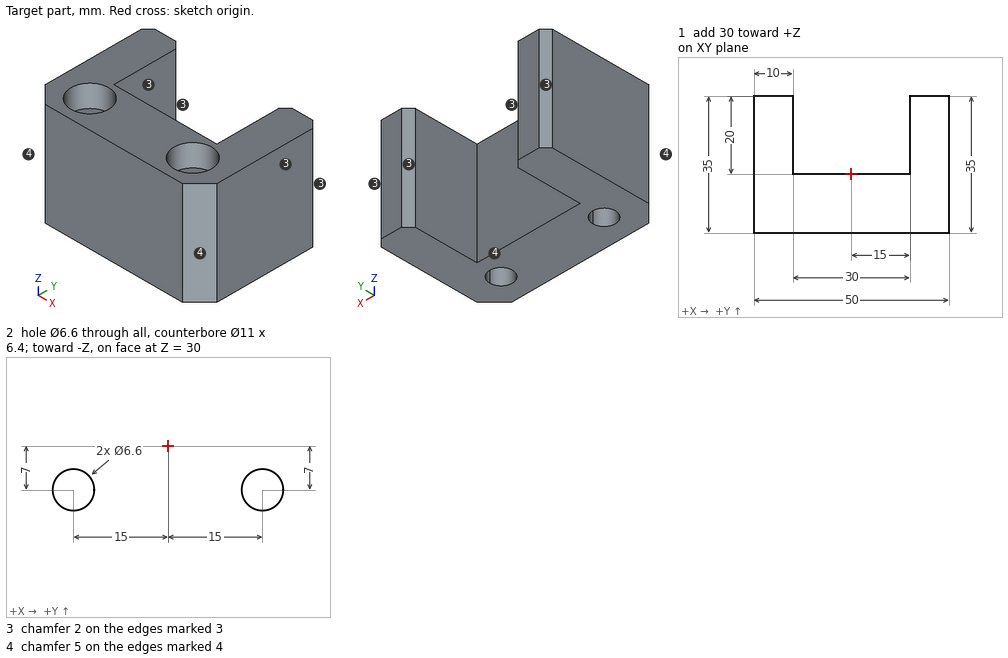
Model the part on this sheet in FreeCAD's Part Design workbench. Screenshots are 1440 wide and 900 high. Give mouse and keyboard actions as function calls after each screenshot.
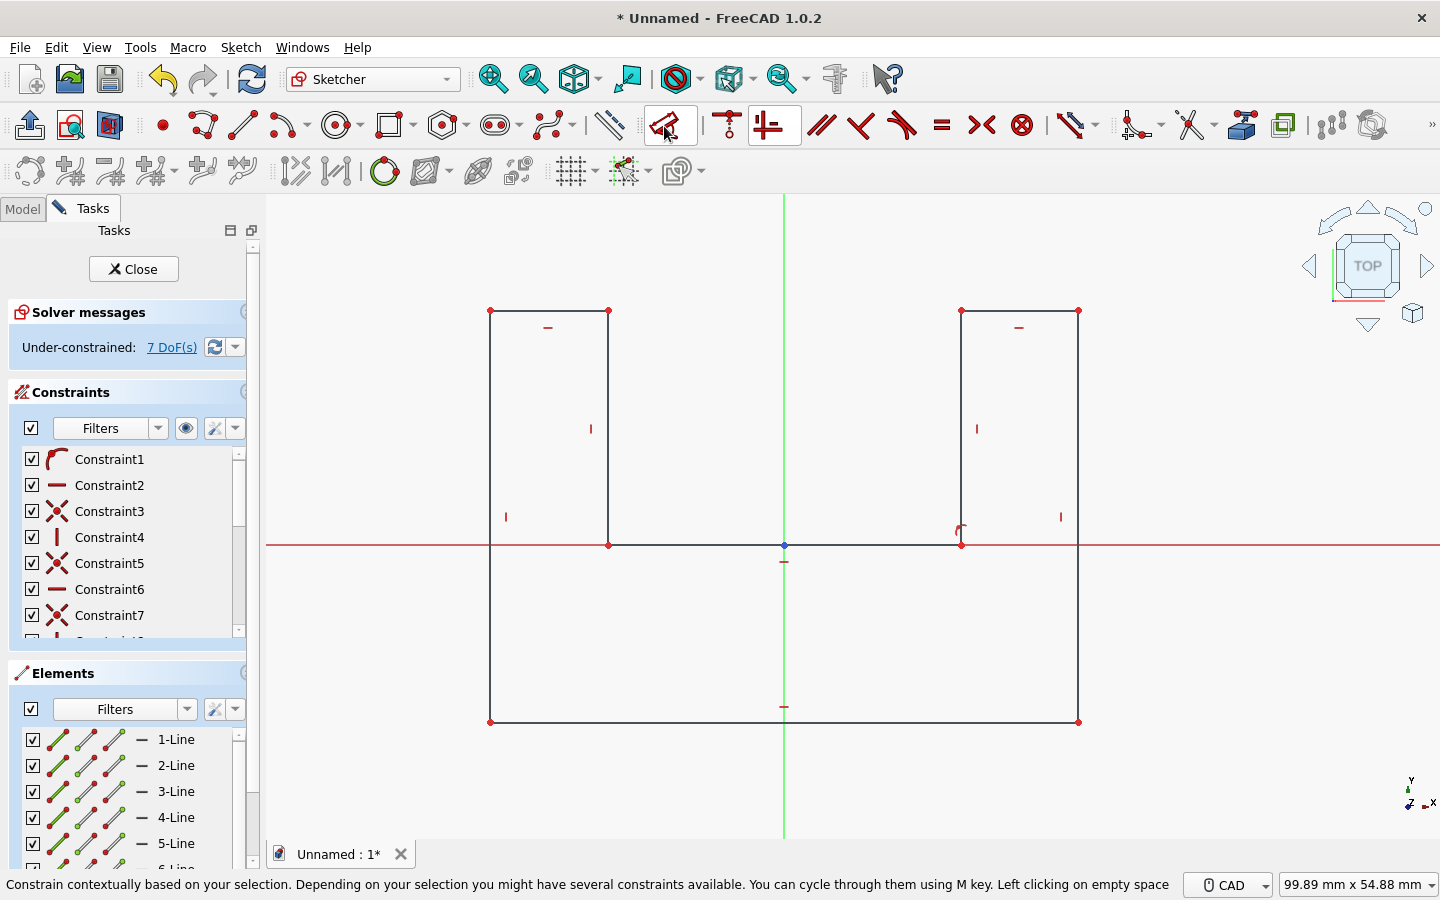
click(855, 545)
click(703, 579)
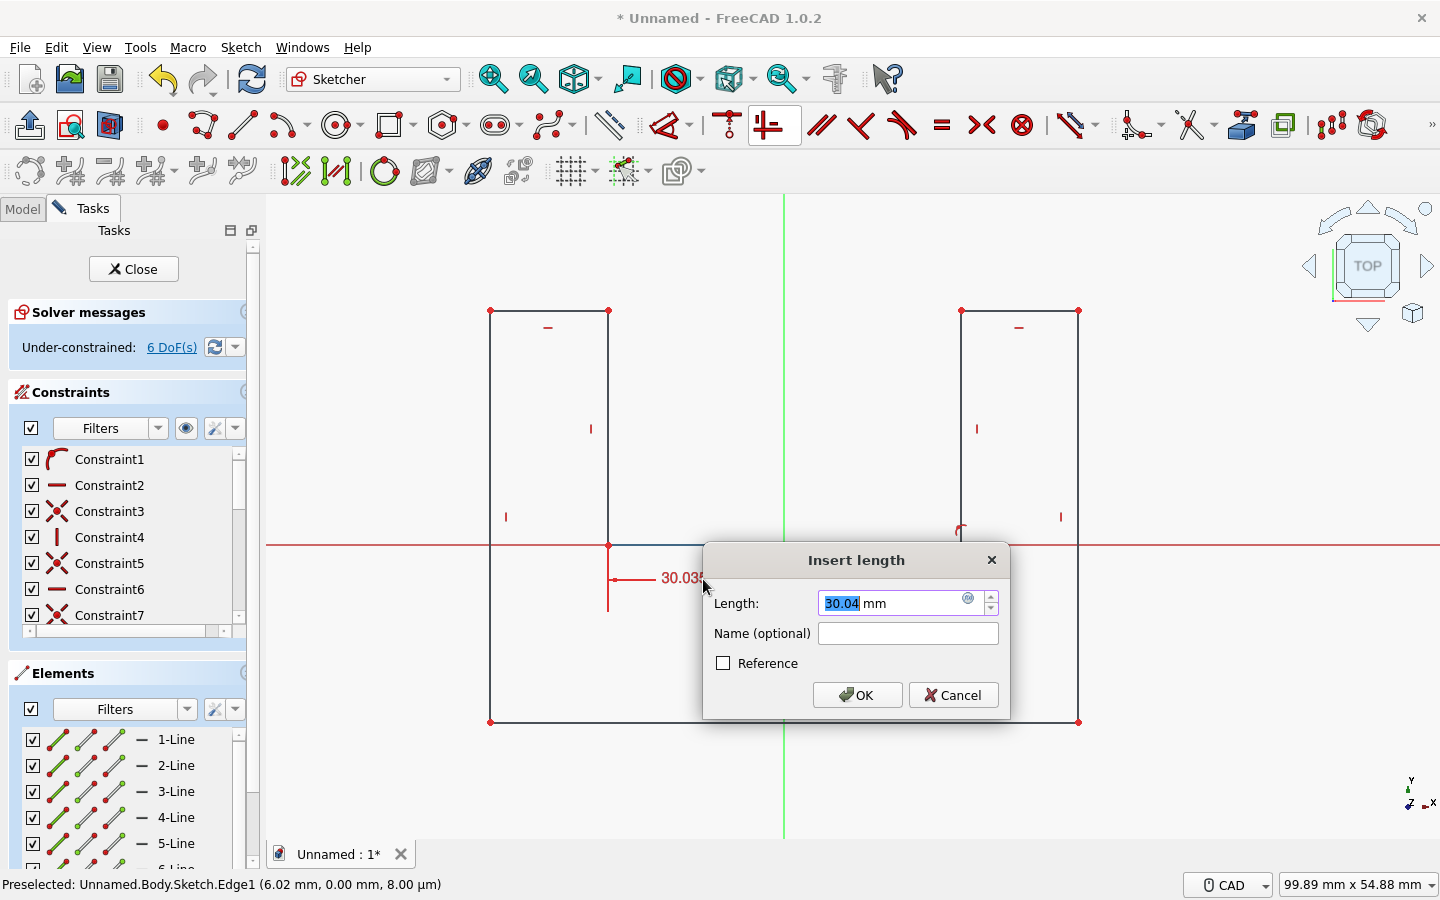
text(30)
key(Return)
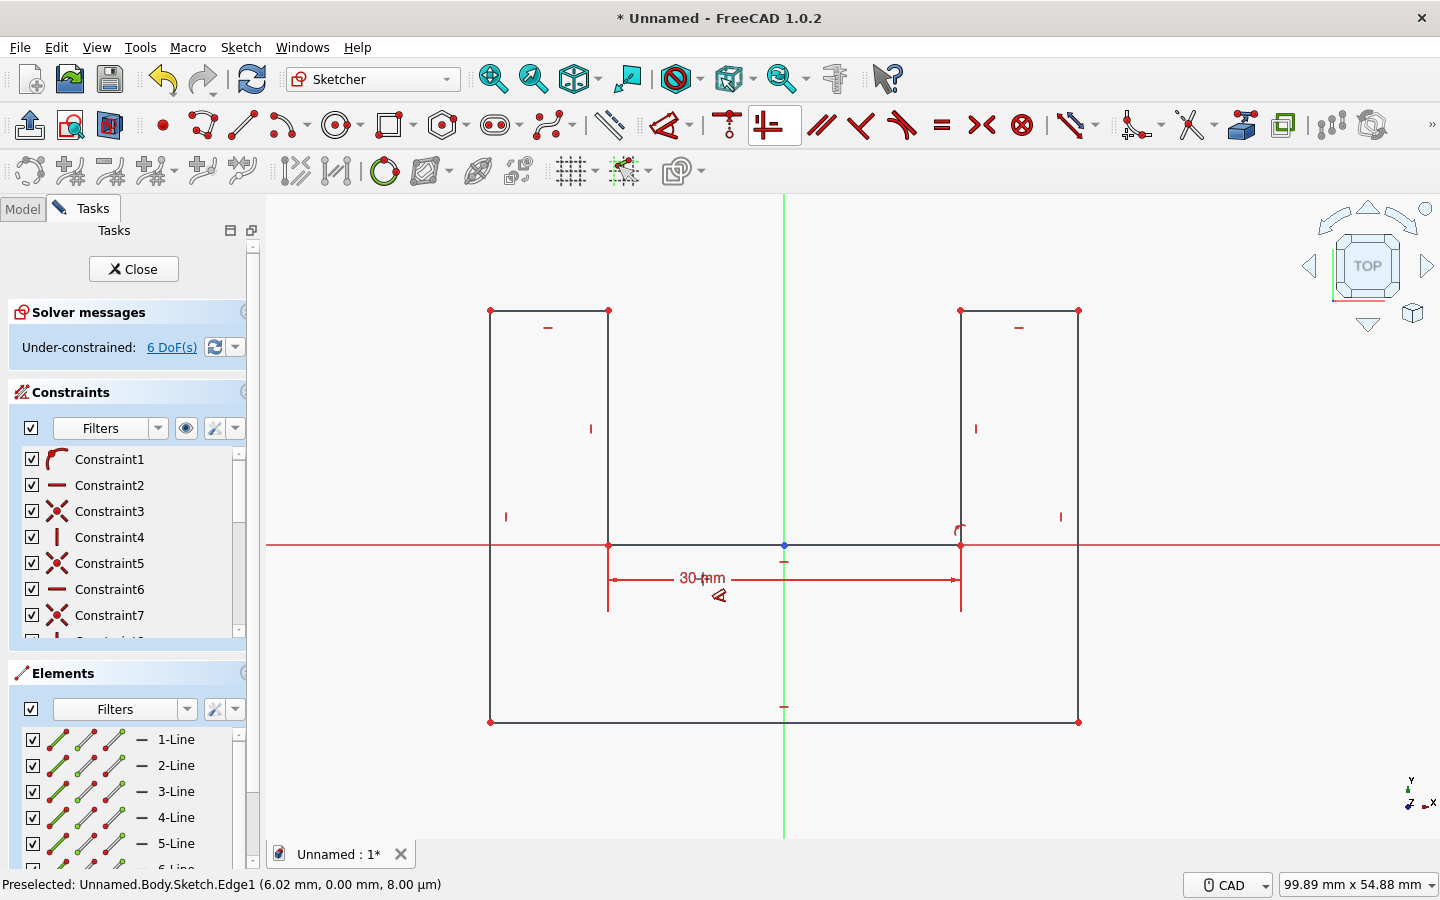
click(608, 475)
click(574, 428)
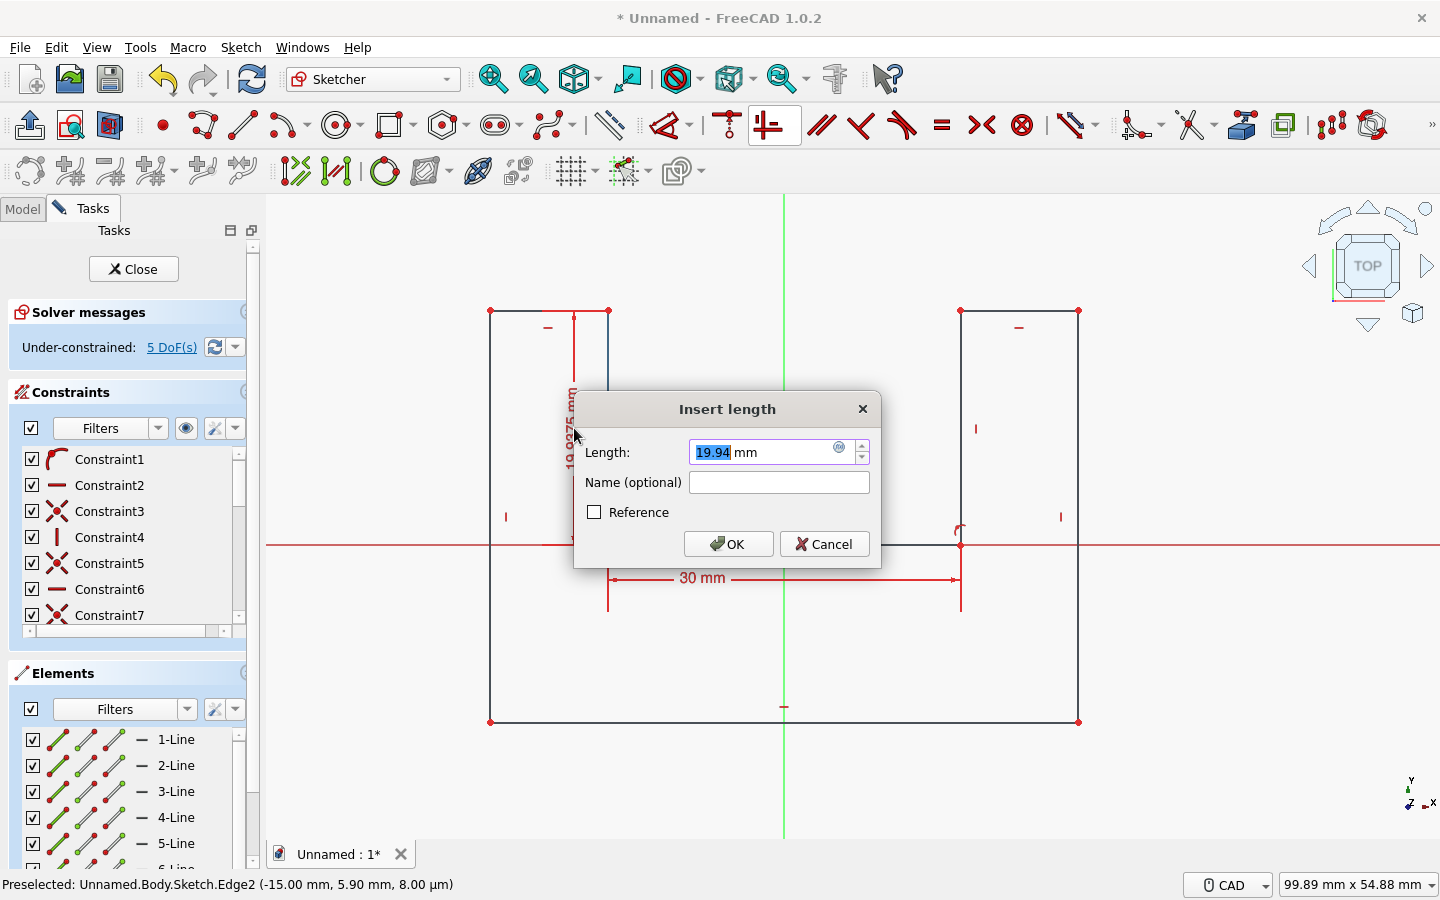
text(20)
key(Return)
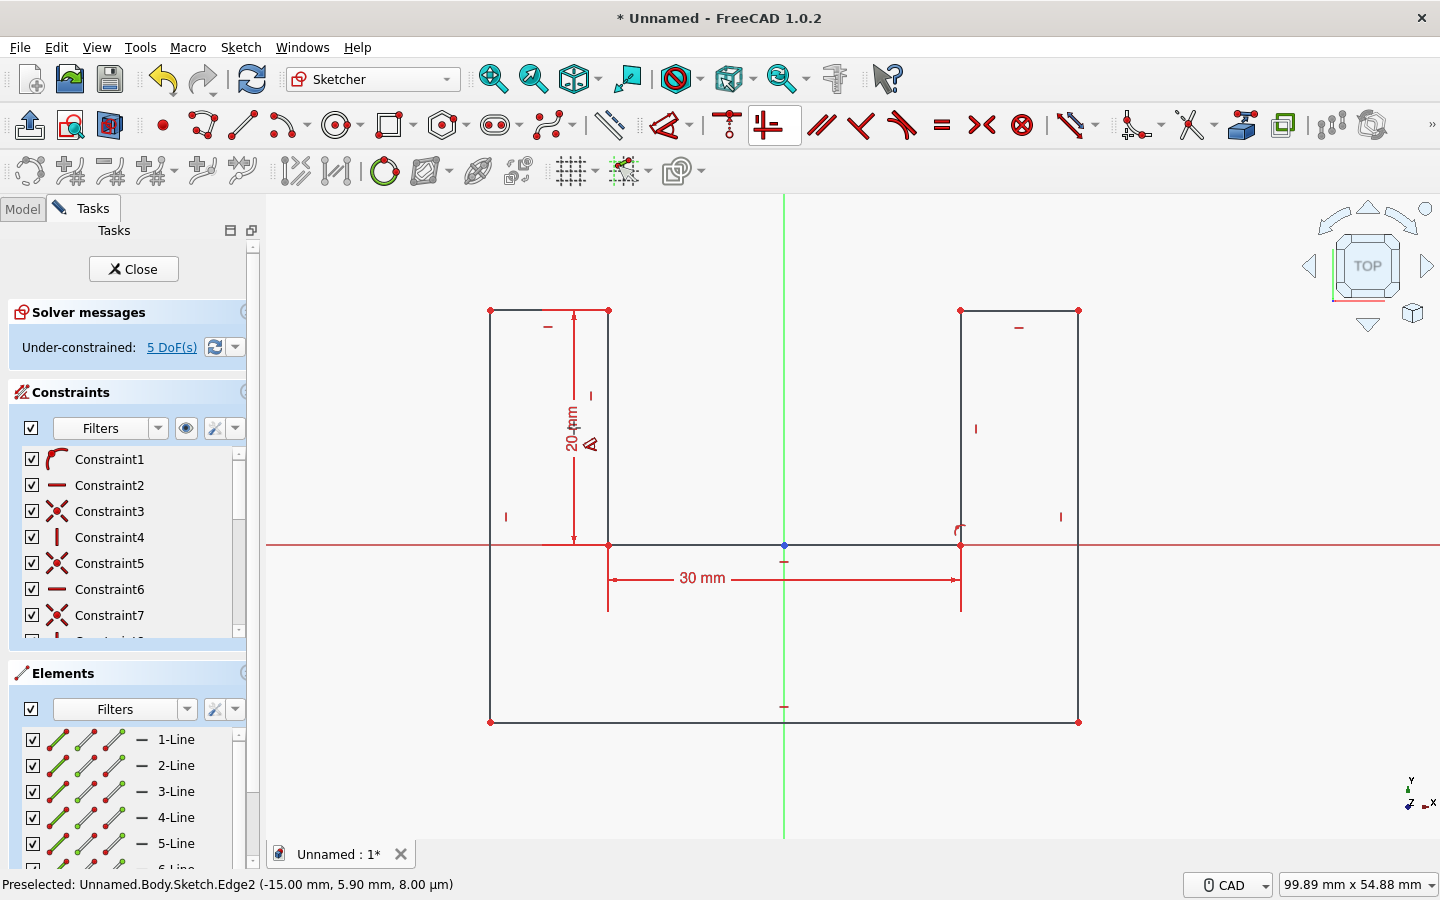
click(573, 310)
click(549, 276)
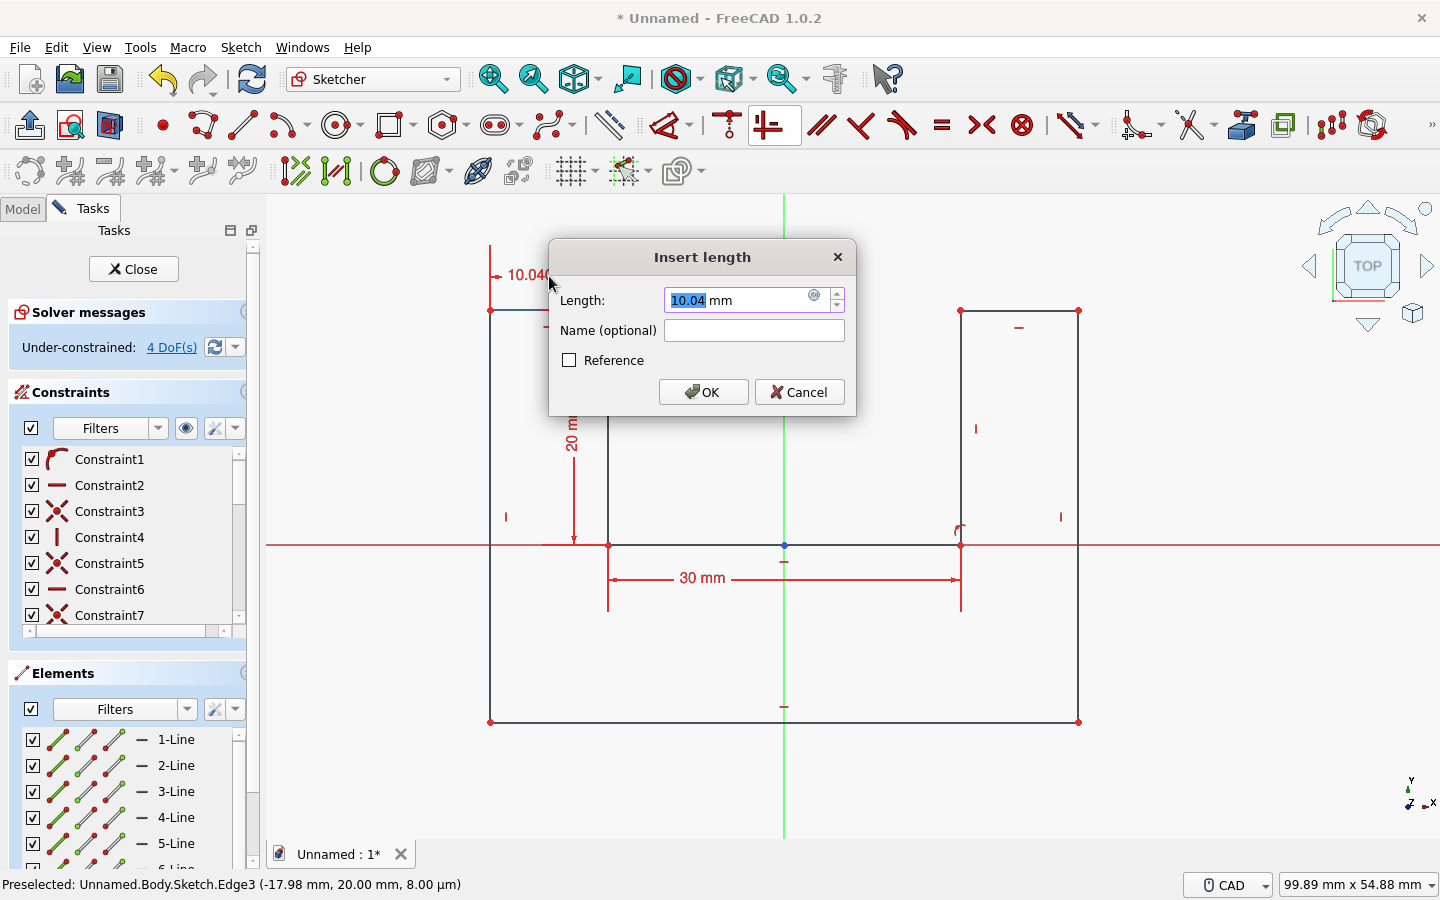
text(10)
key(Return)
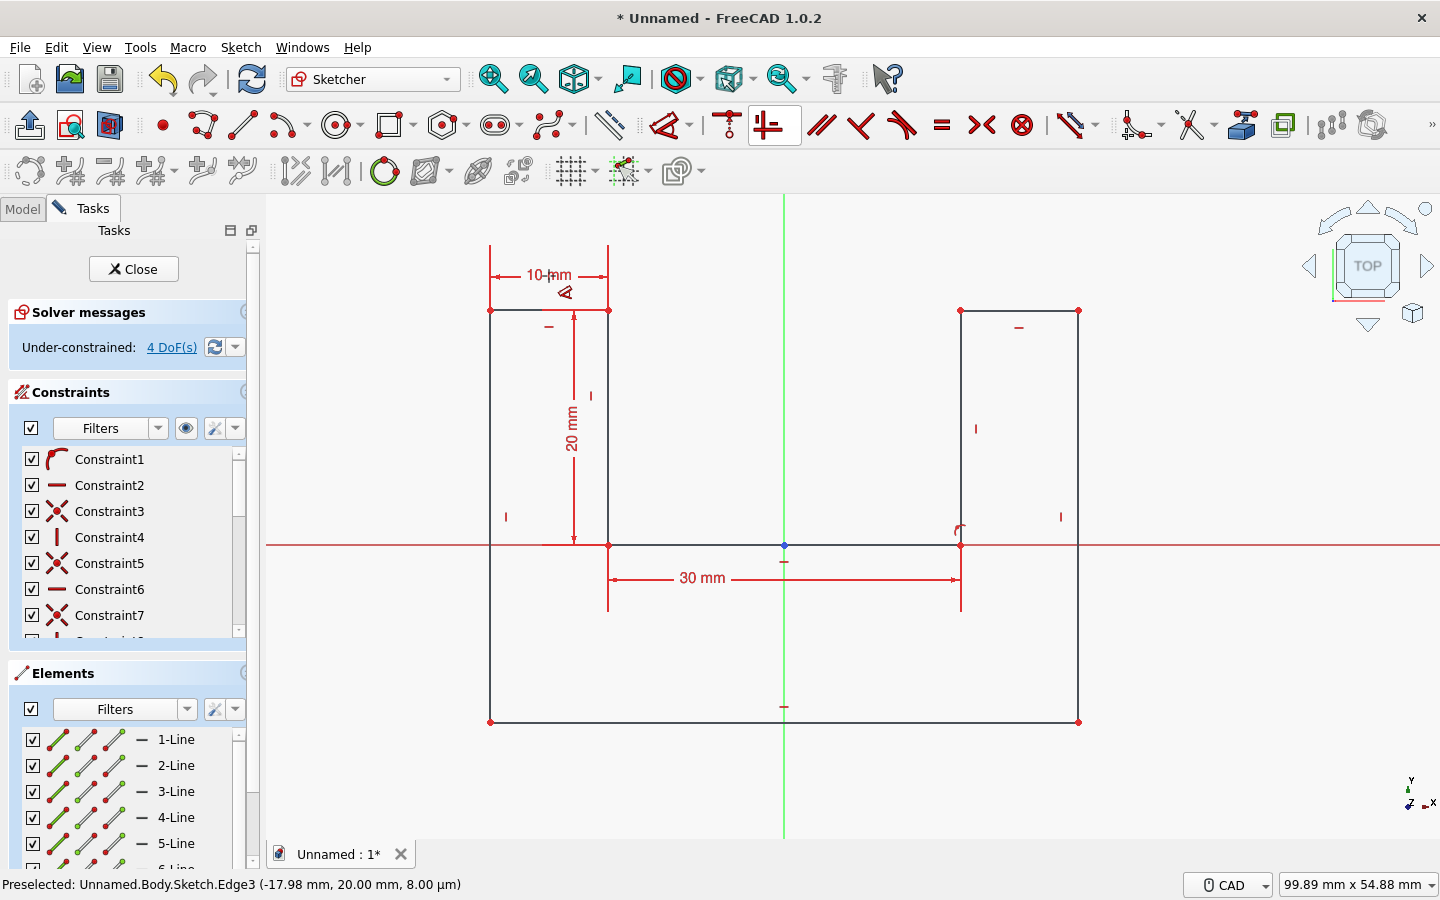
click(490, 434)
click(456, 517)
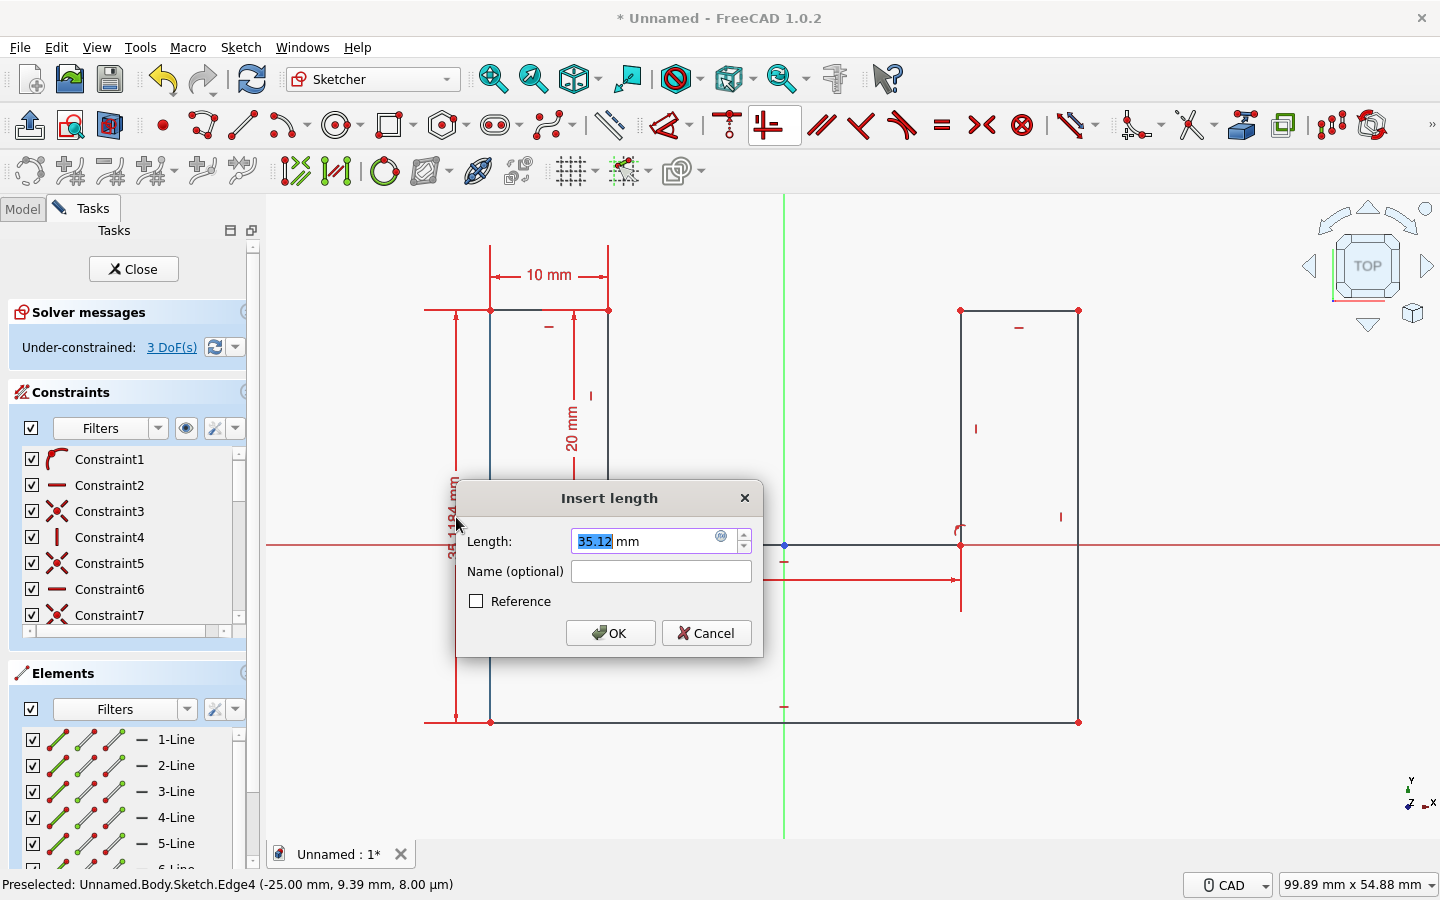
text(35)
key(Return)